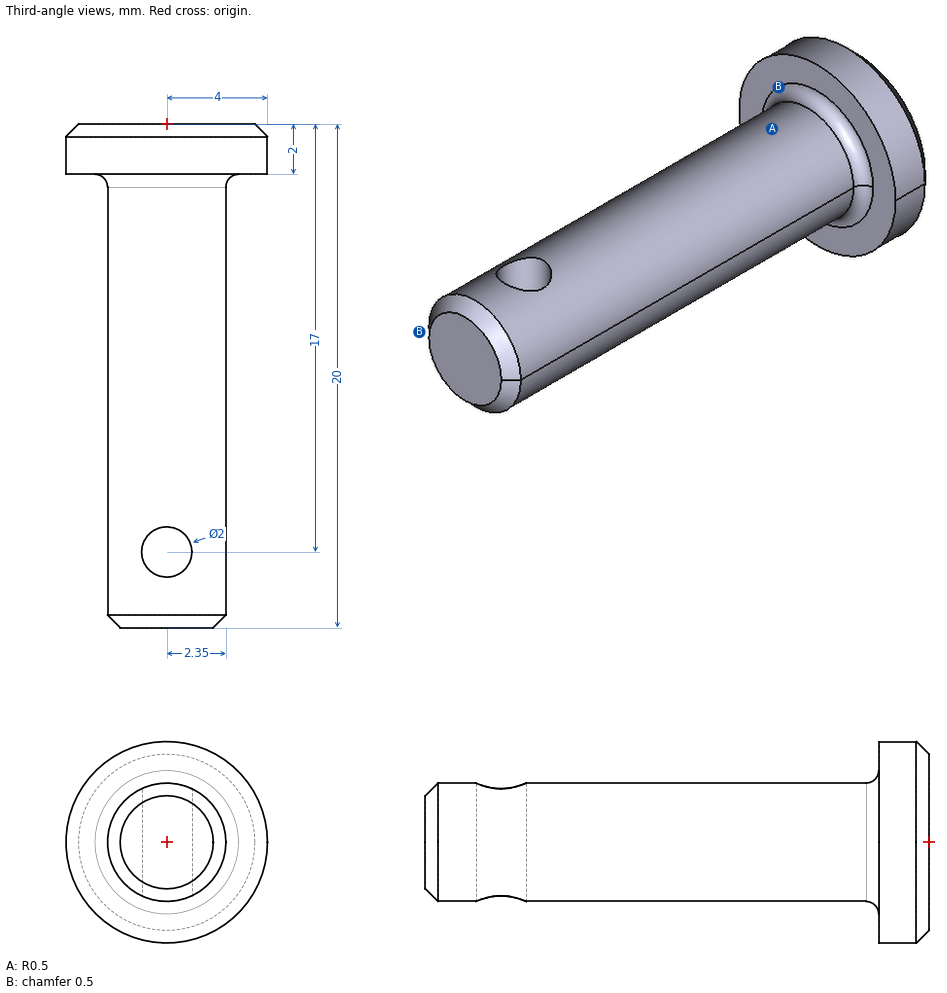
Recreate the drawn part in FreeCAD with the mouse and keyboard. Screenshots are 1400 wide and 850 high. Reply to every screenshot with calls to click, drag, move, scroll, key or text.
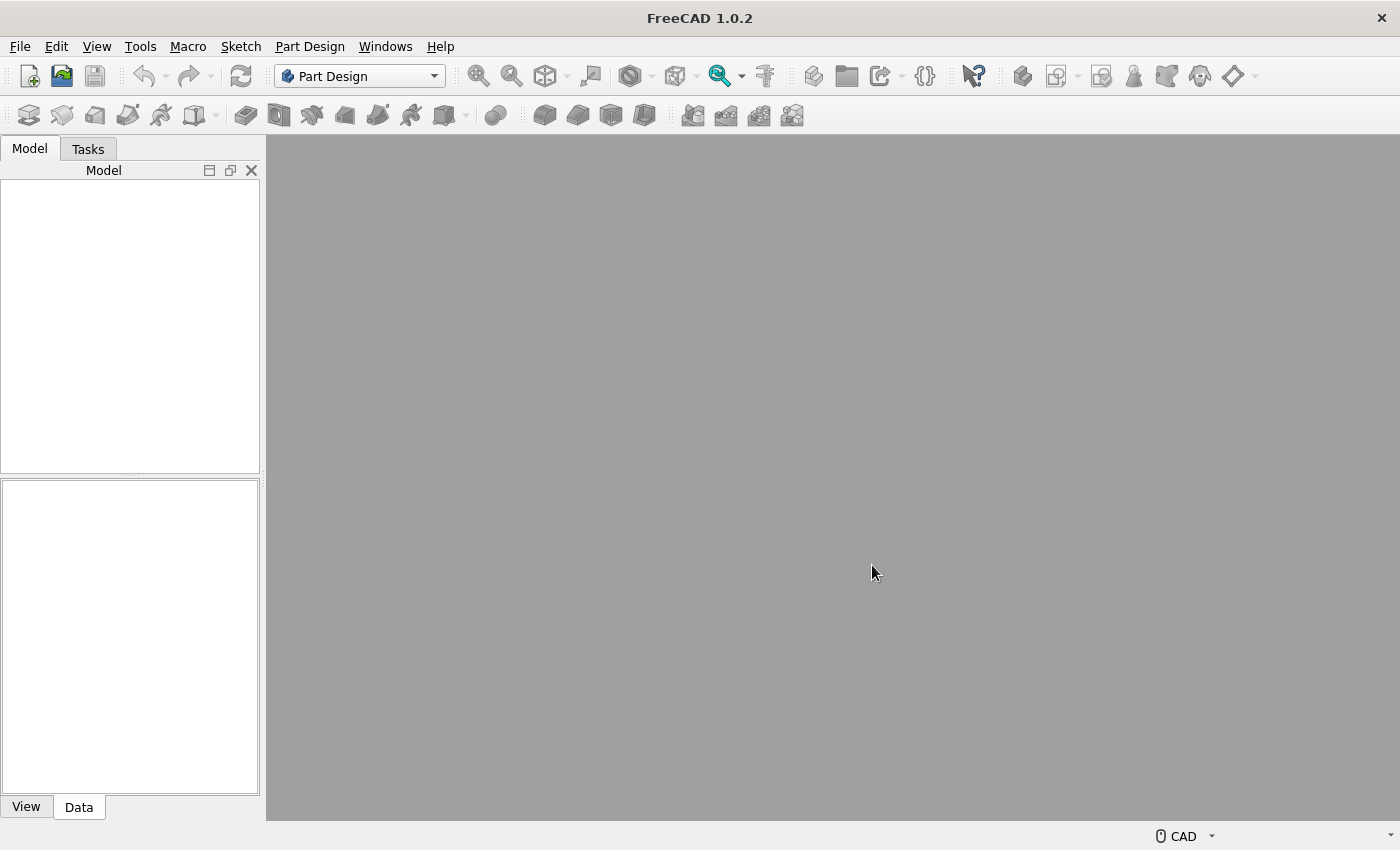
key(ctrl+n)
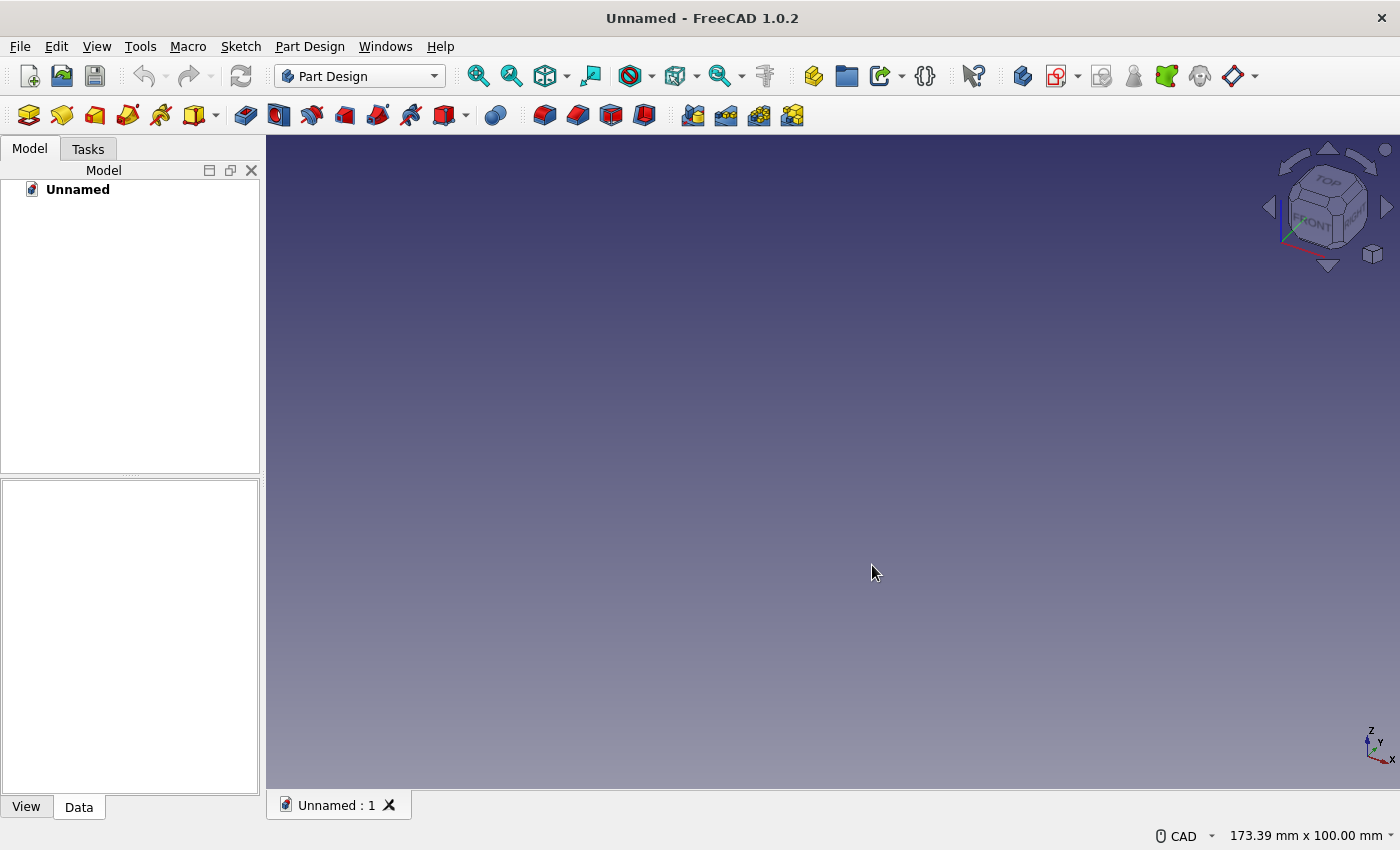
click(1056, 76)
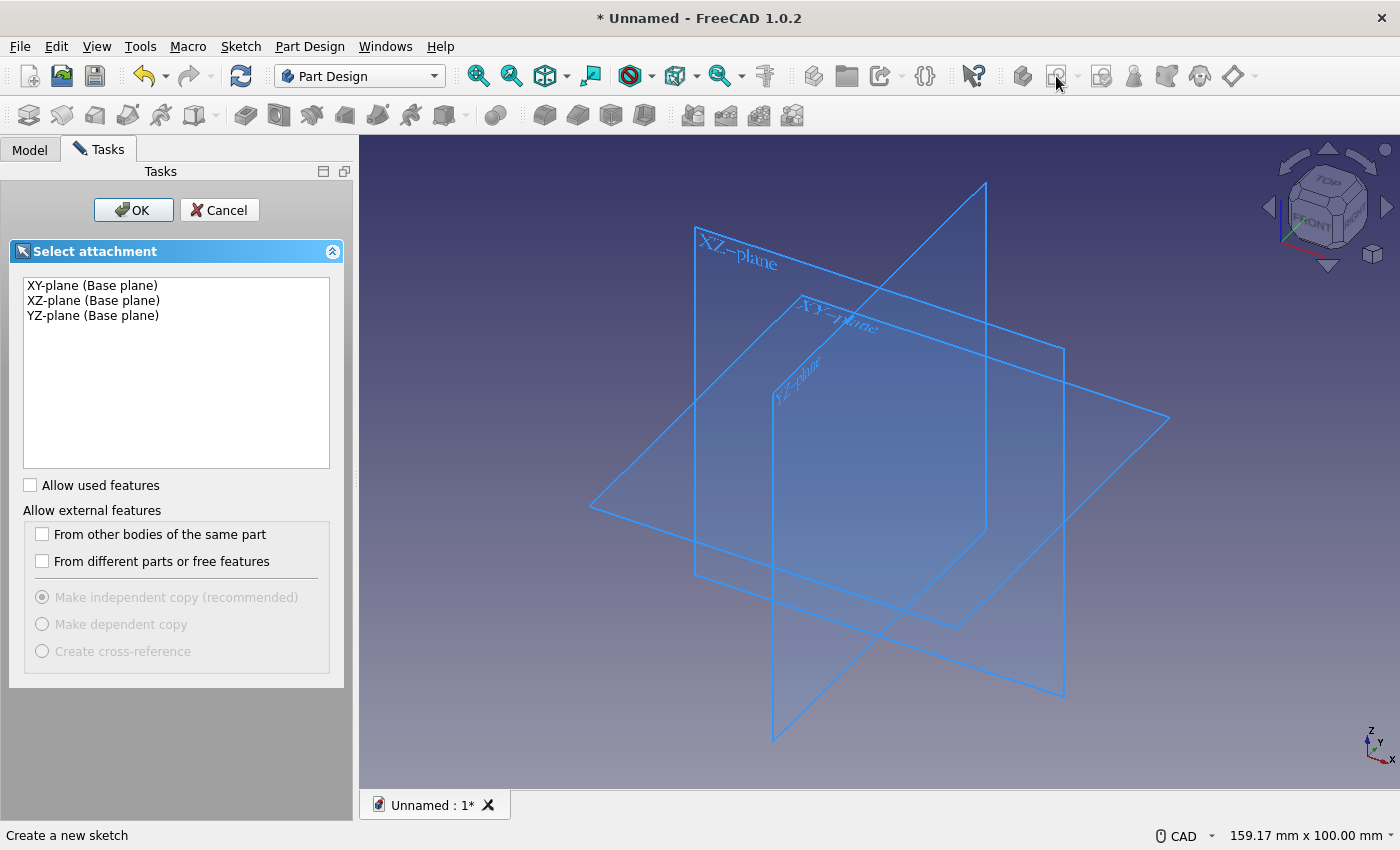
click(84, 286)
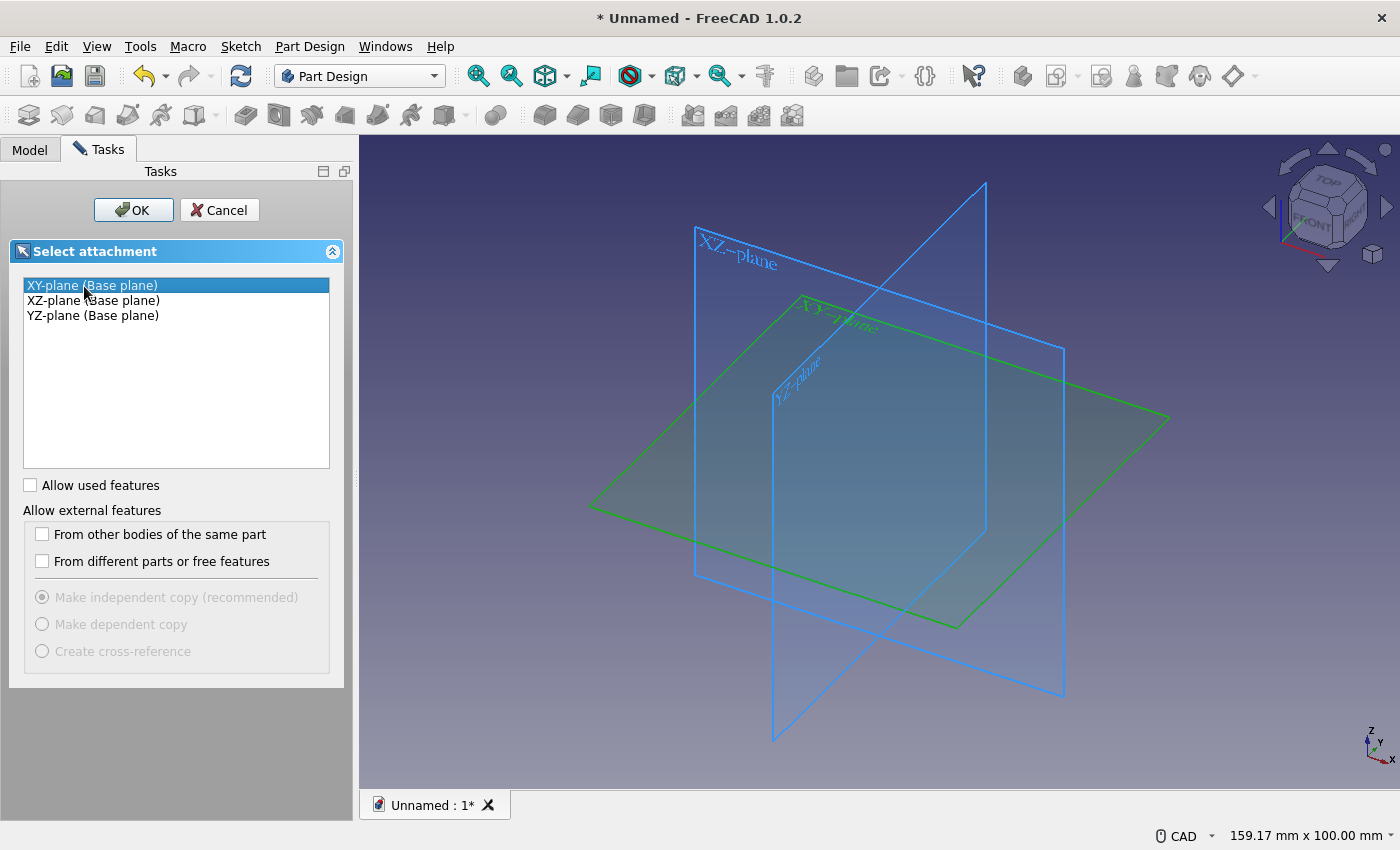
click(134, 210)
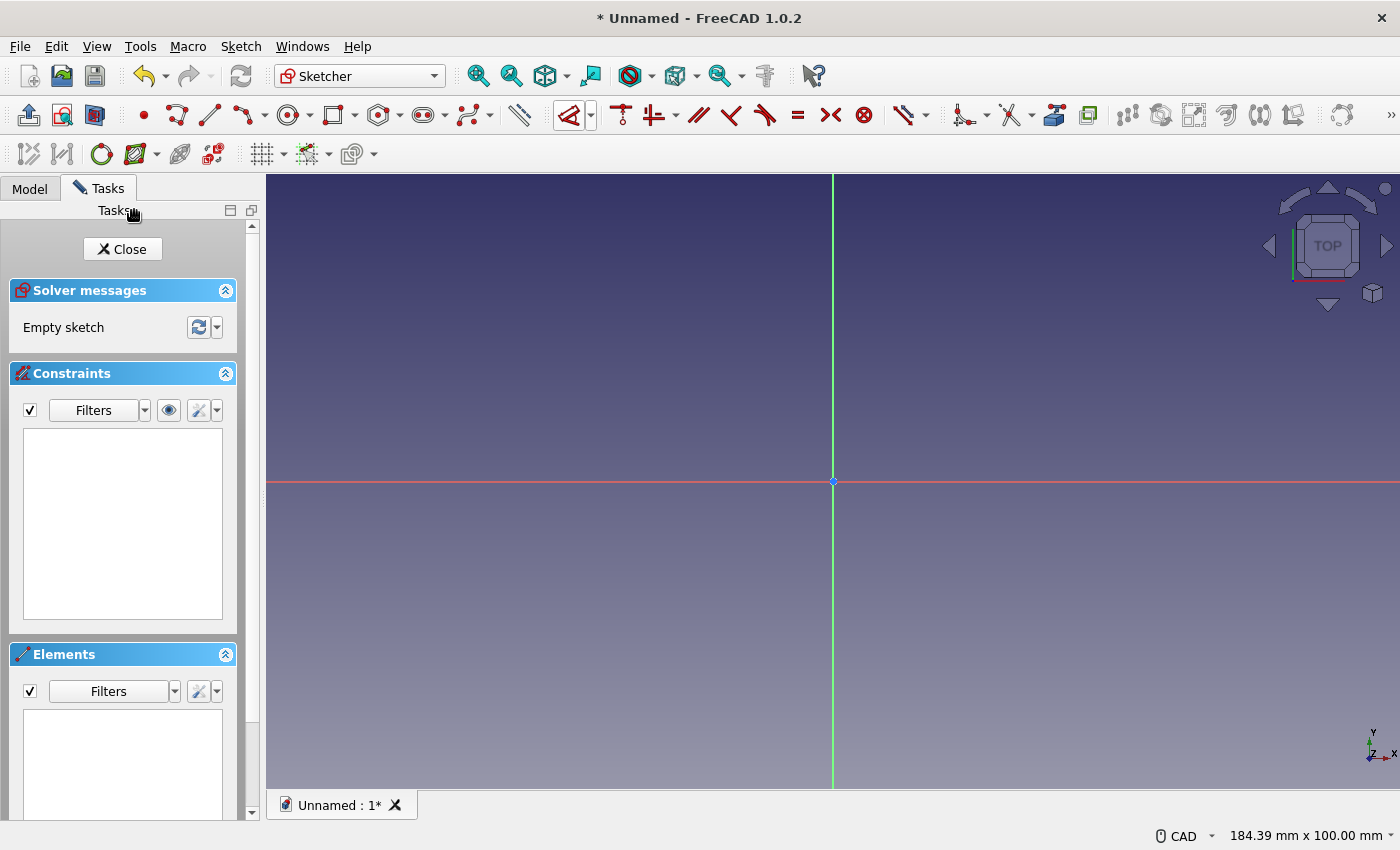
scroll(880, 570, up, 6)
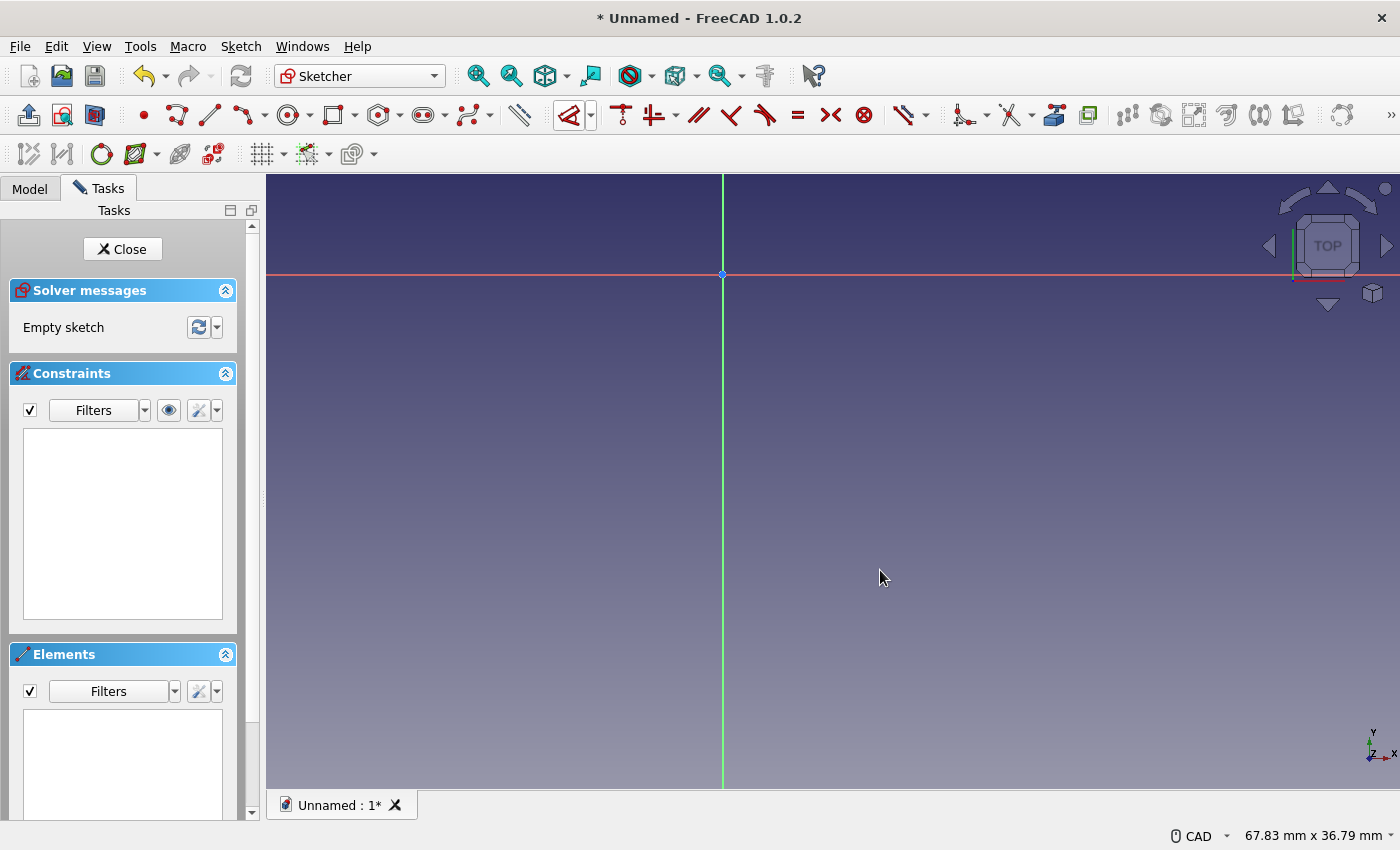
click(177, 116)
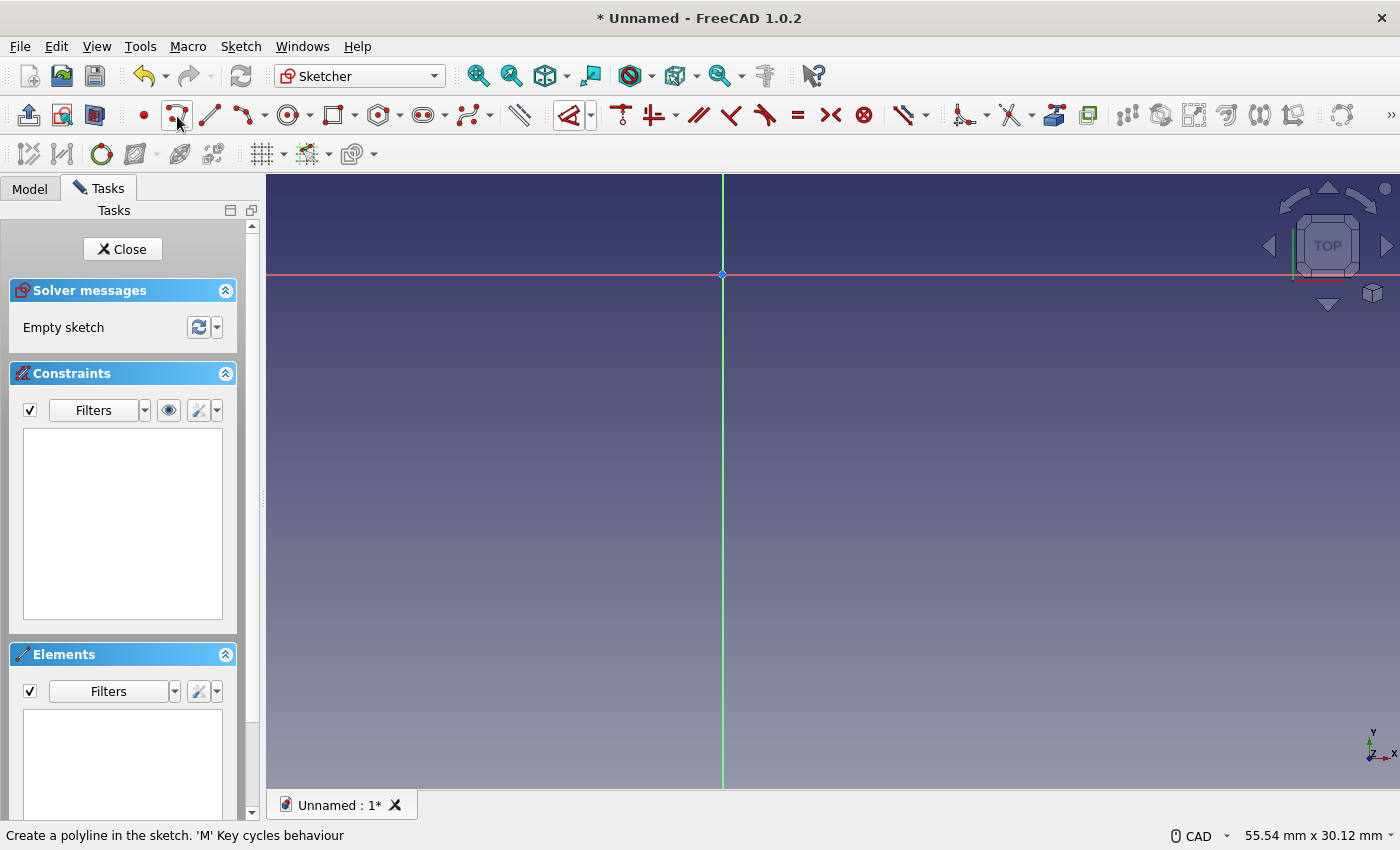
click(723, 275)
click(732, 683)
click(771, 683)
click(771, 316)
click(804, 316)
click(804, 284)
click(723, 275)
key(Escape)
key(Escape)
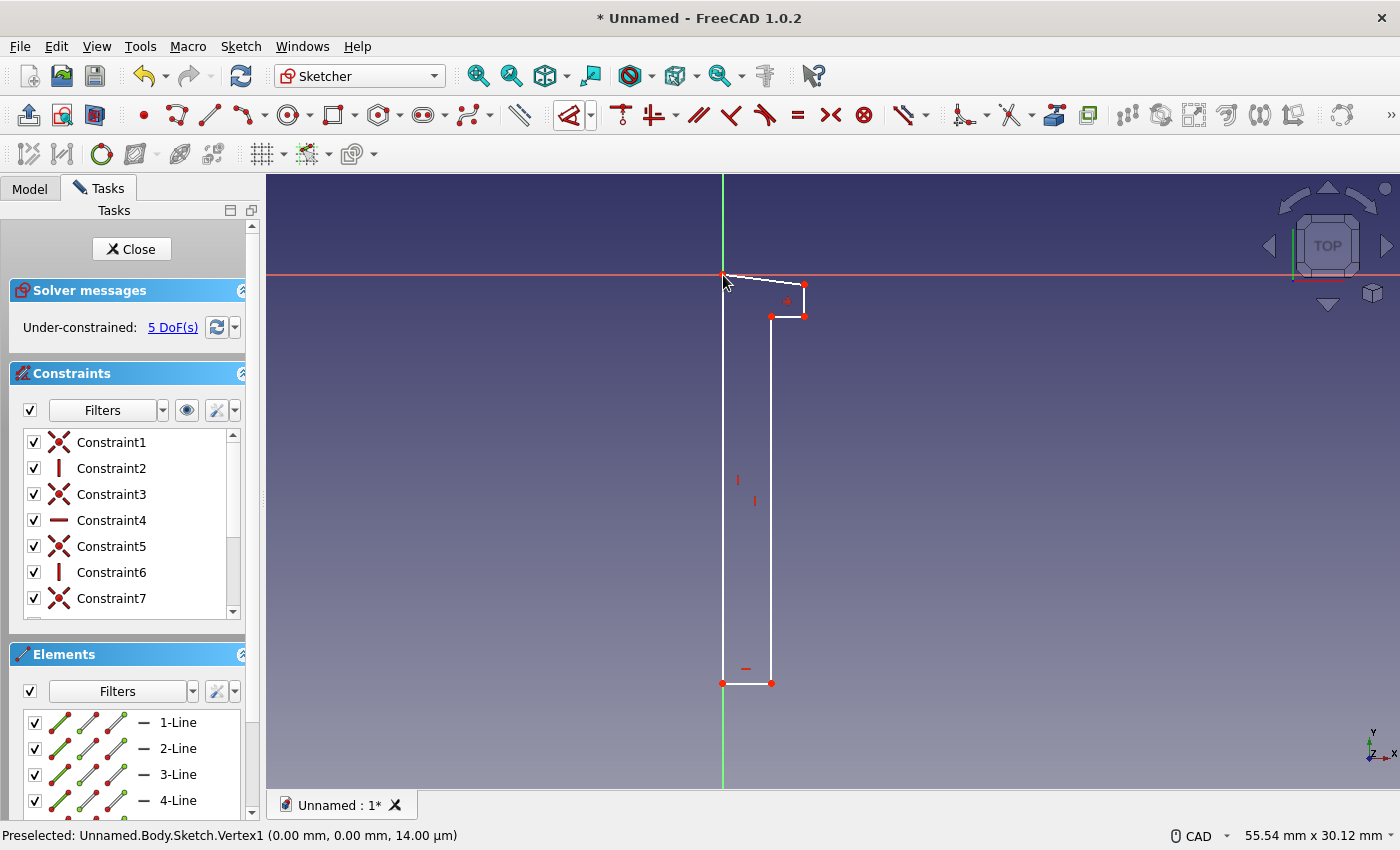
click(747, 278)